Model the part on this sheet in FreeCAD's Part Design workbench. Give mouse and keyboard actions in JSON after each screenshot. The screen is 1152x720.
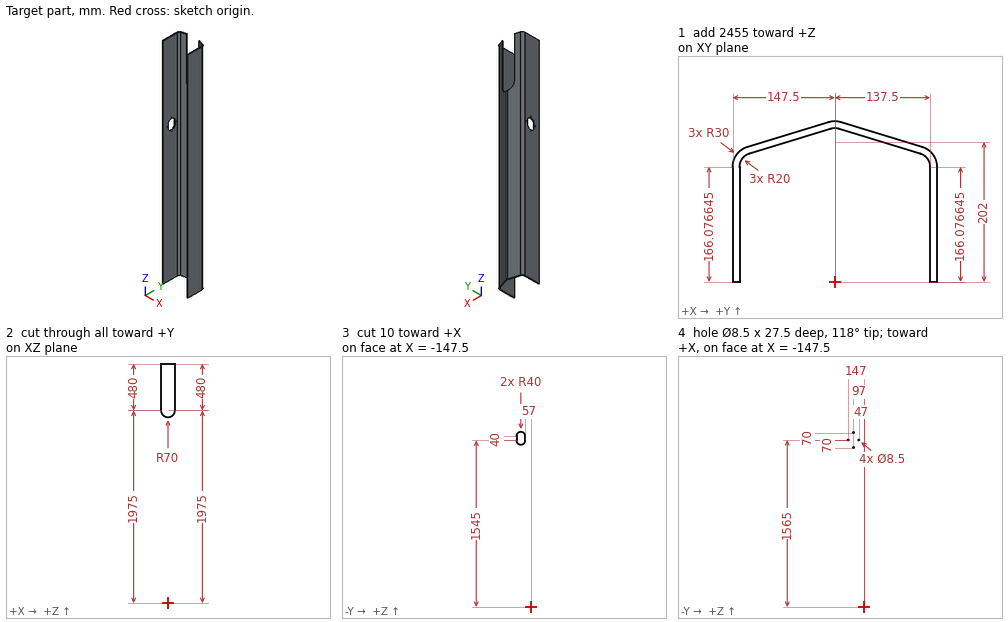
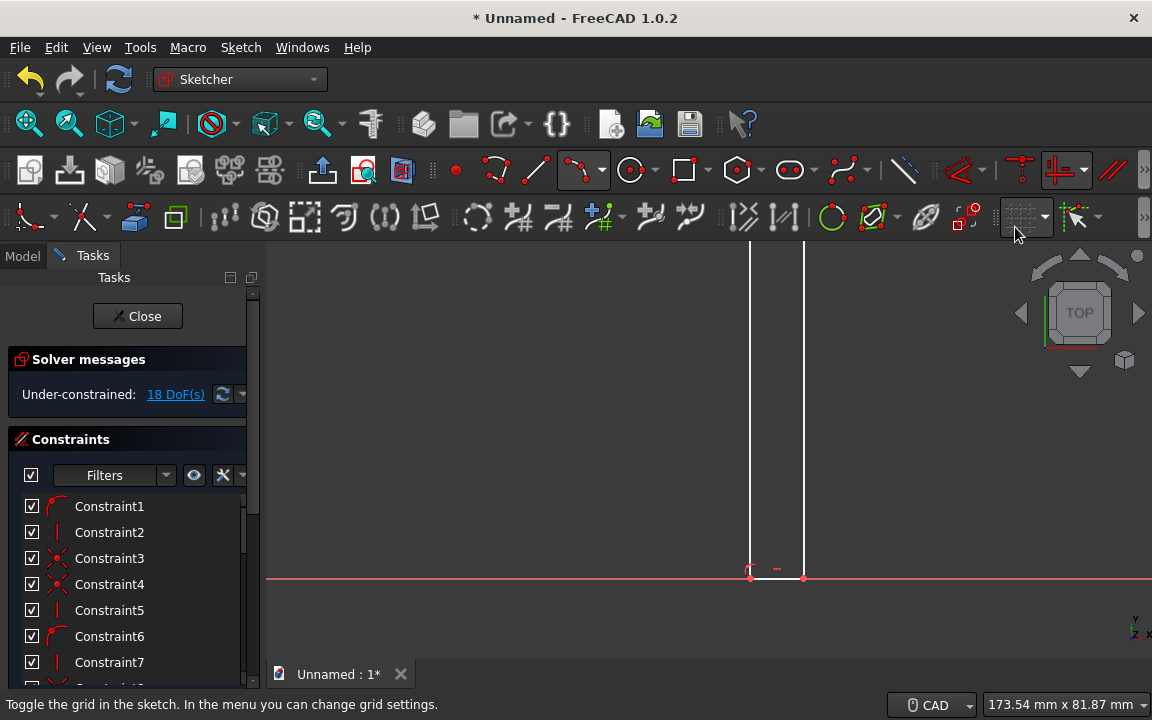
{"action": "scroll", "coordinate": [791, 567], "scroll_direction": "down", "scroll_amount": 8}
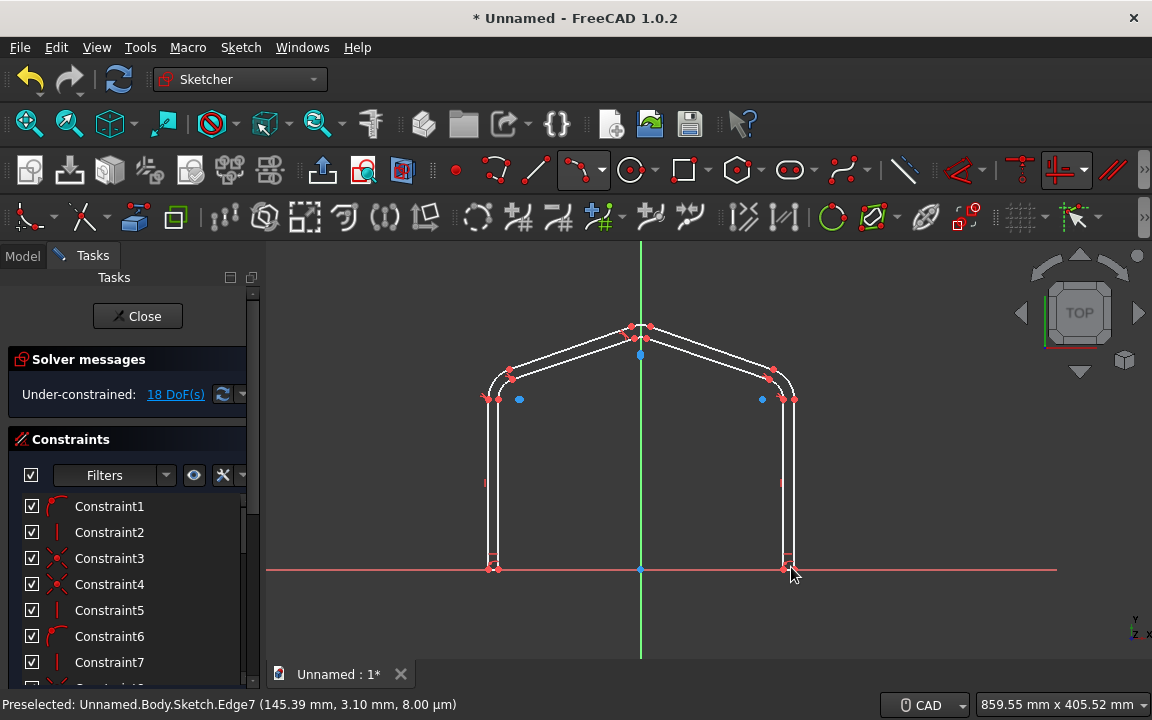
{"action": "scroll", "coordinate": [782, 392], "scroll_direction": "up", "scroll_amount": 3}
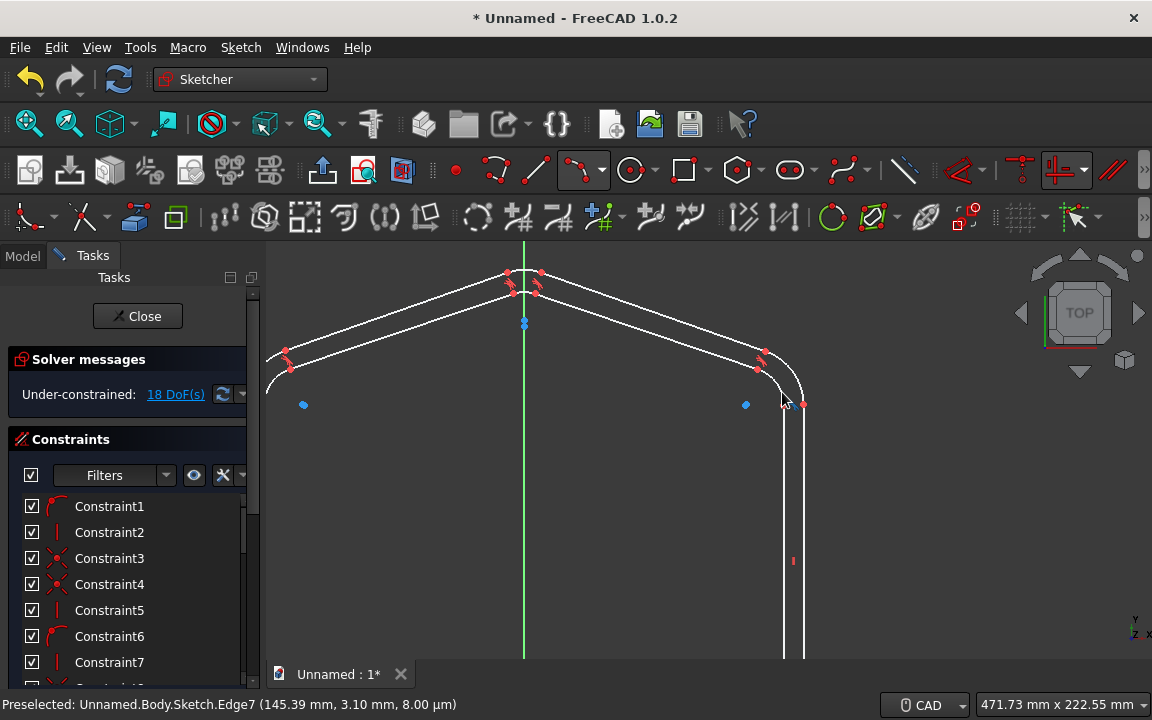
{"action": "left_click", "coordinate": [781, 392]}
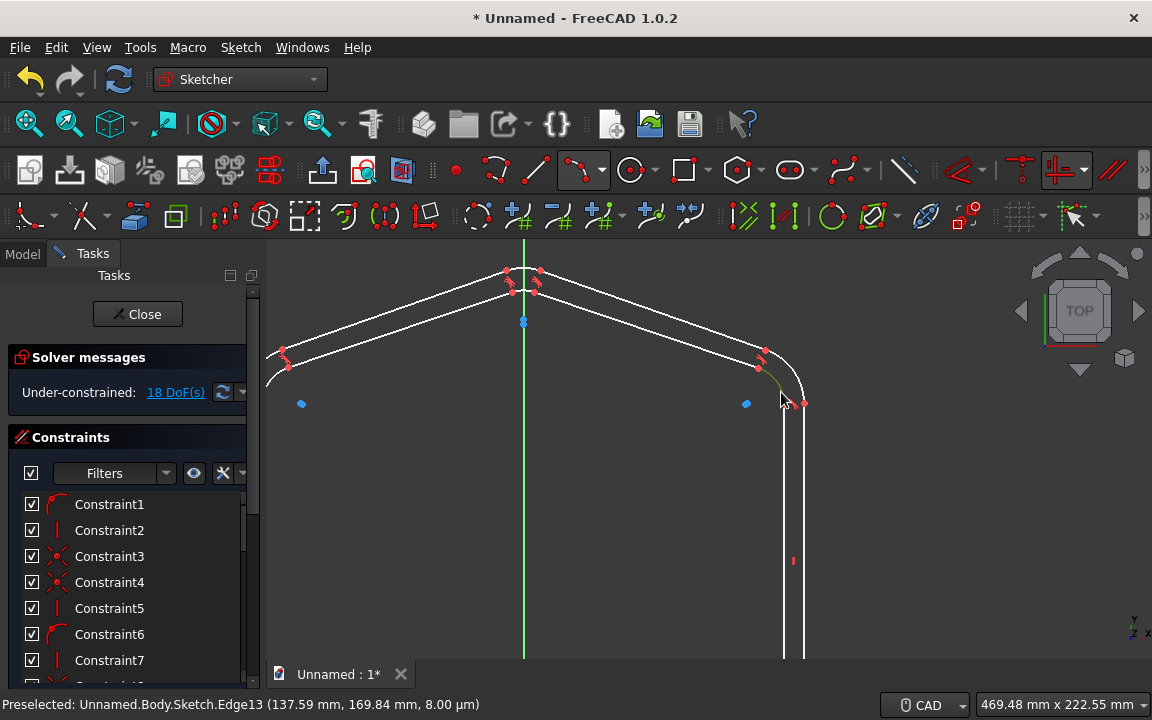
{"action": "left_click", "coordinate": [800, 383]}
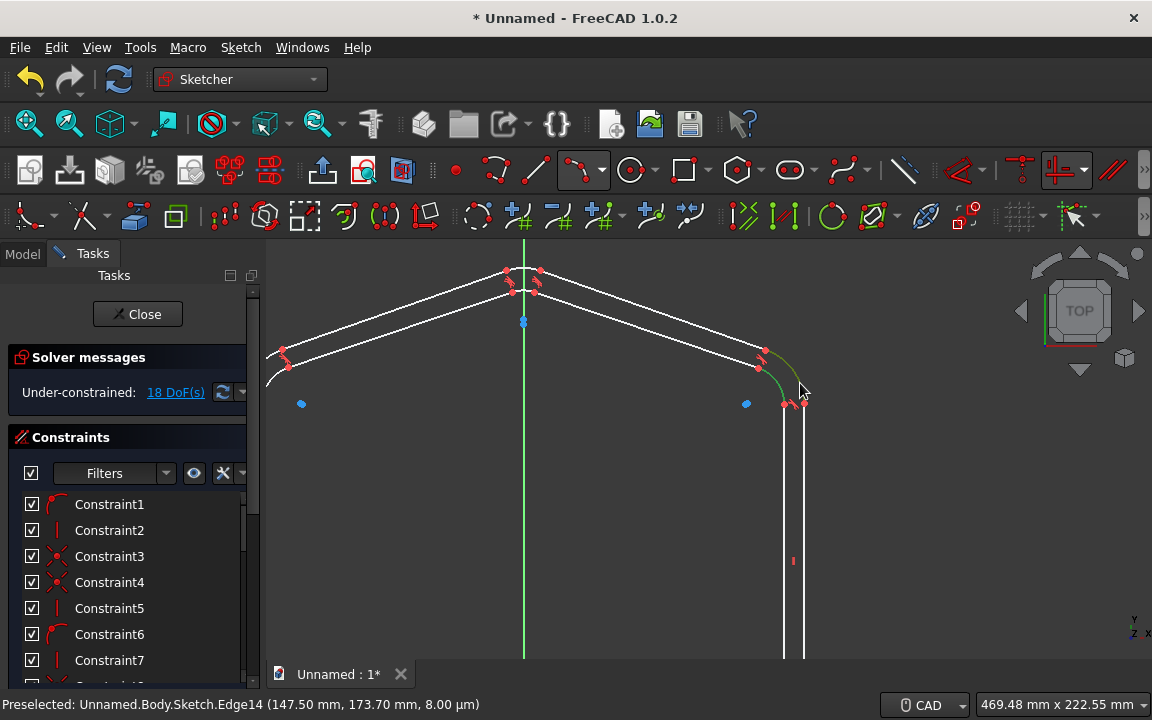
{"action": "left_click", "coordinate": [1020, 170]}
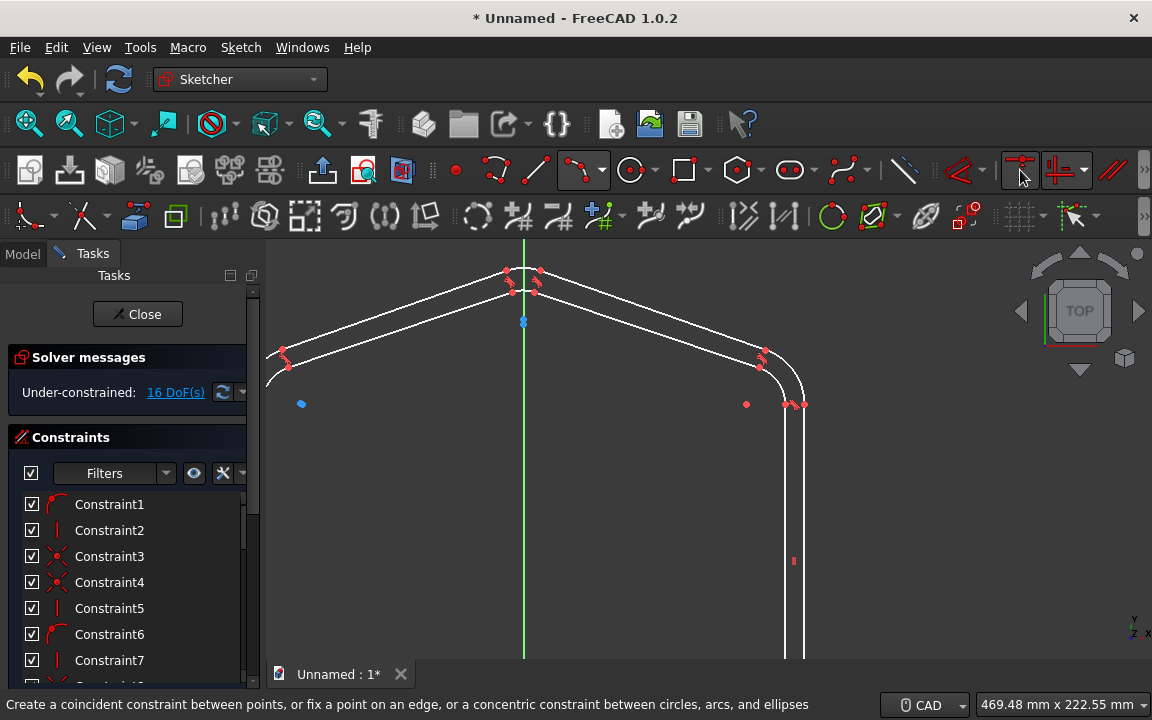
{"action": "scroll", "coordinate": [523, 290], "scroll_direction": "up", "scroll_amount": 2}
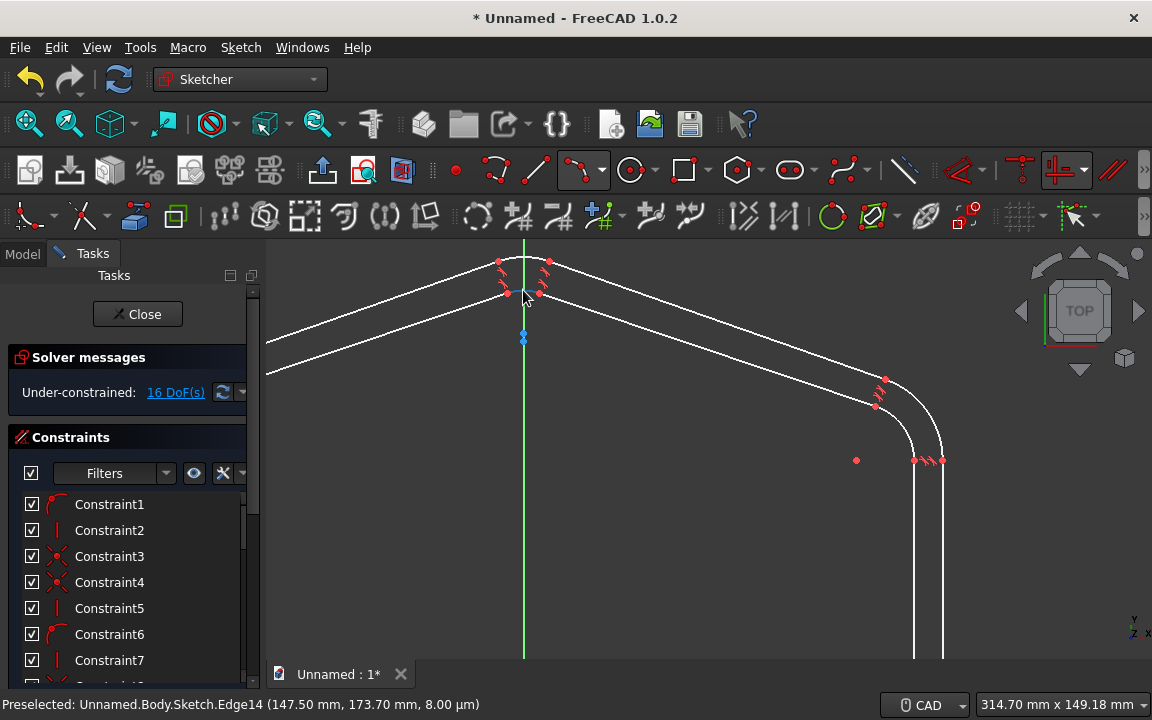
{"action": "left_click", "coordinate": [523, 291]}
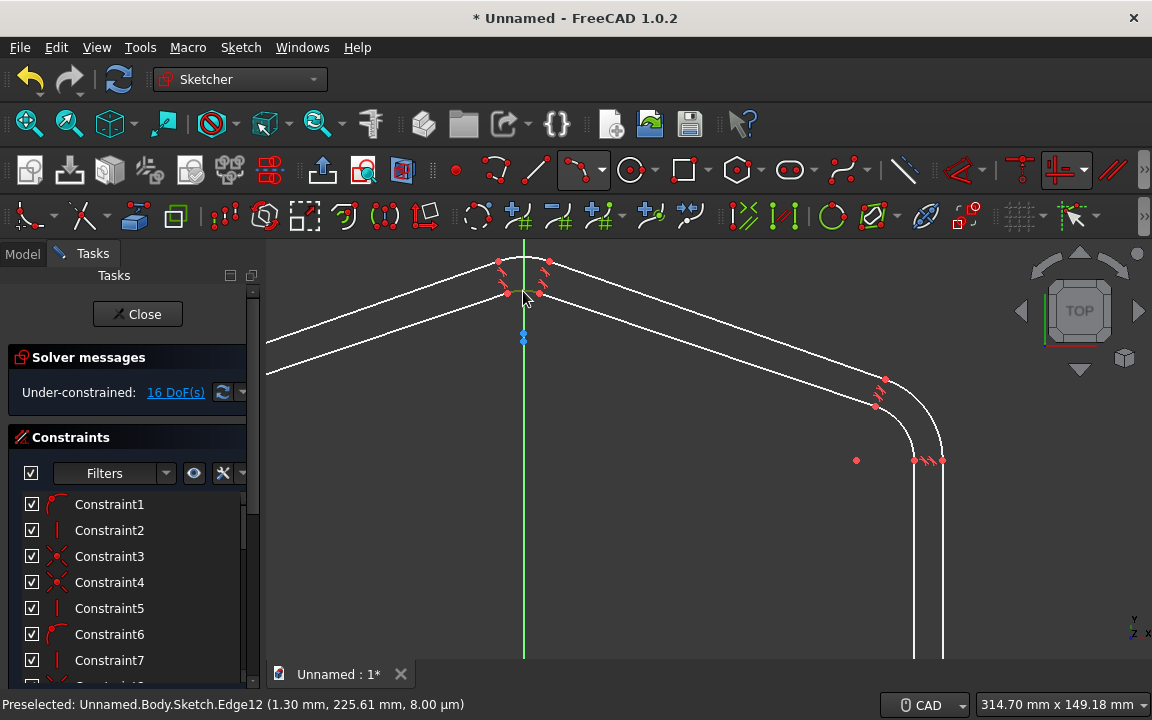
{"action": "scroll", "coordinate": [708, 362], "scroll_direction": "down", "scroll_amount": 5}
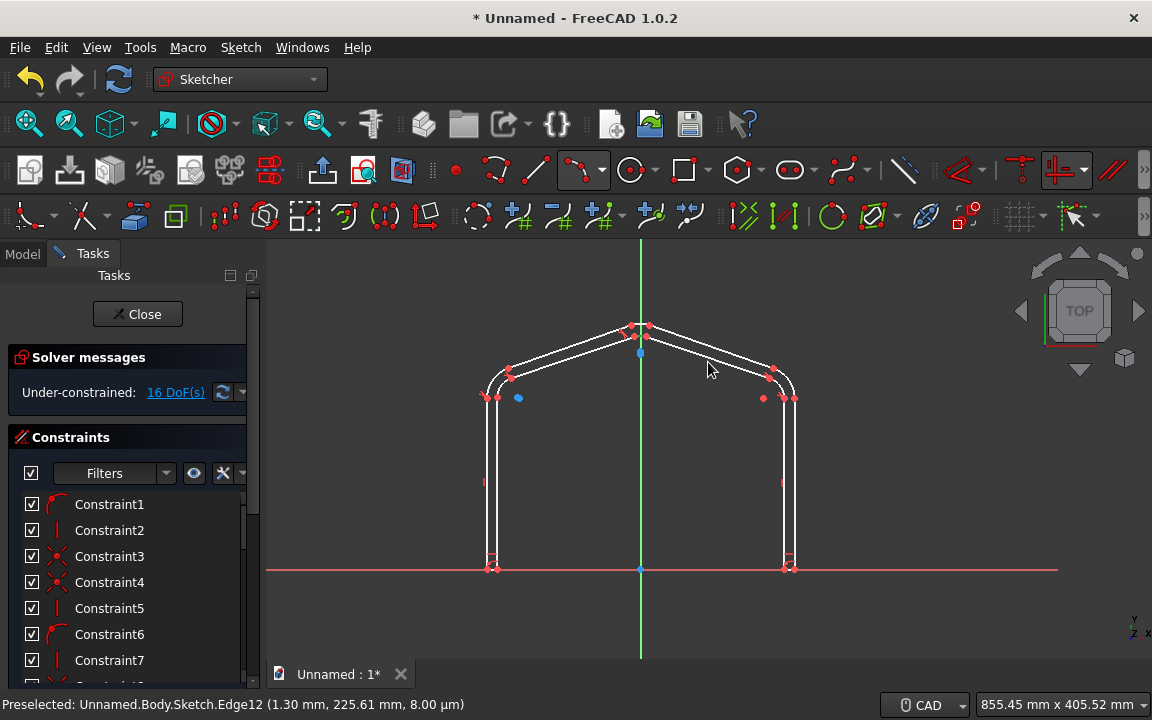
{"action": "scroll", "coordinate": [644, 324], "scroll_direction": "up", "scroll_amount": 7}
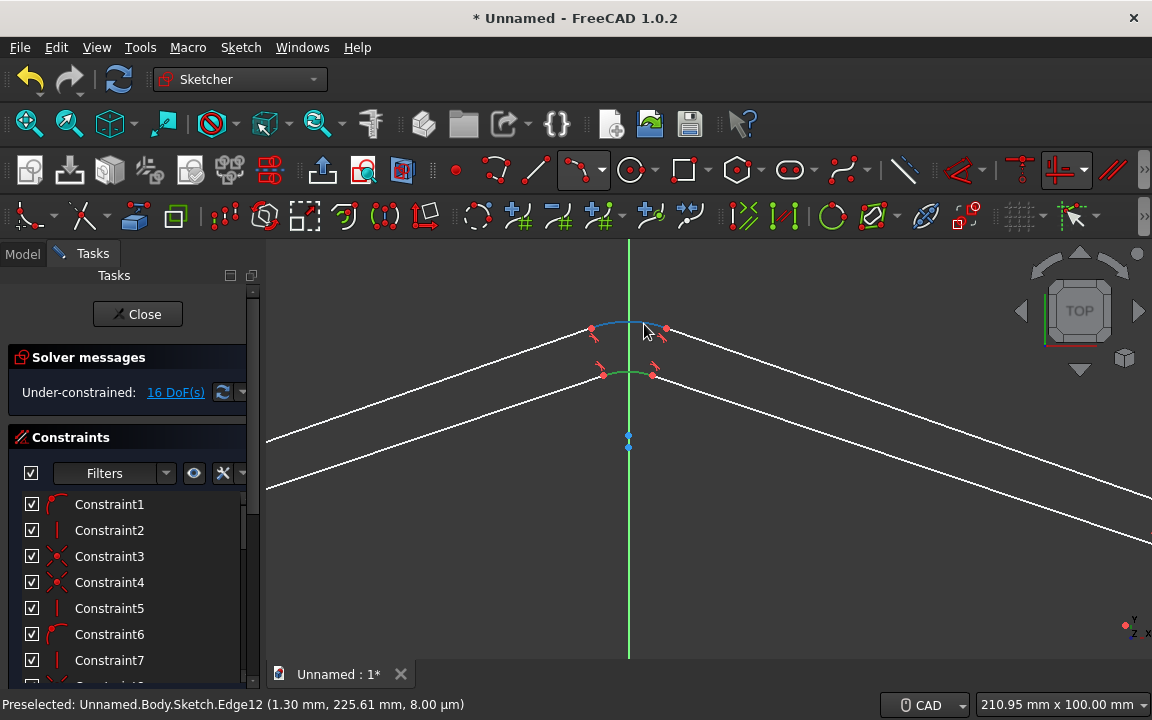
{"action": "left_click", "coordinate": [644, 323]}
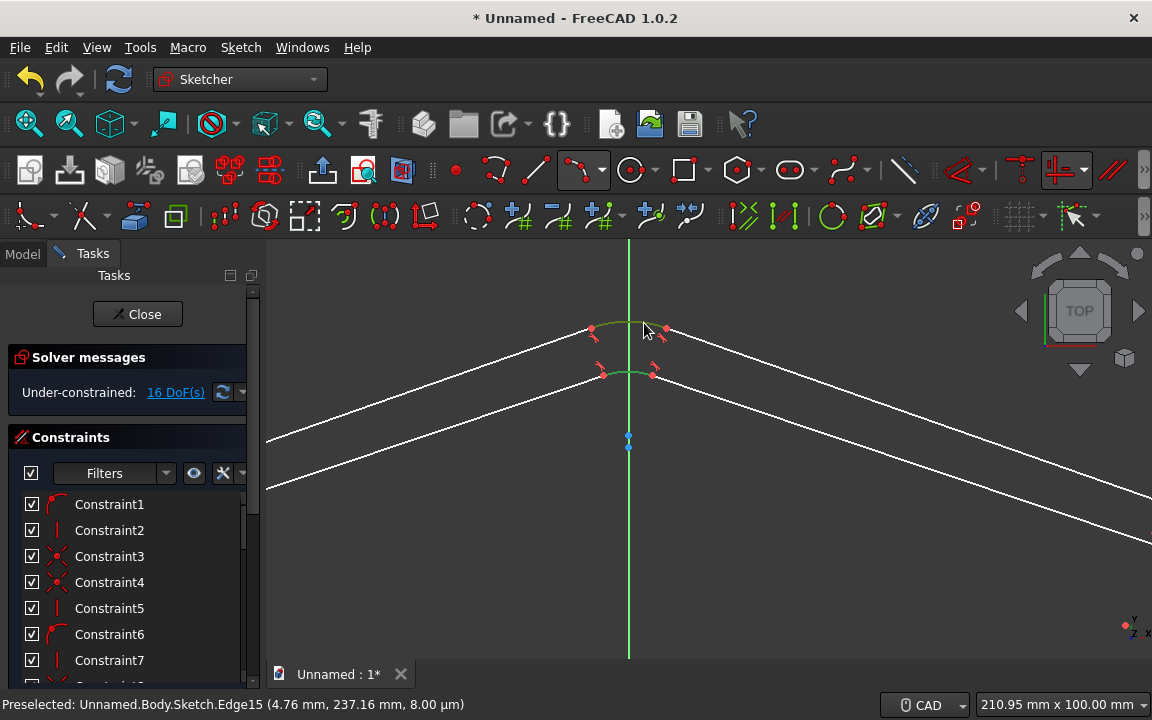
{"action": "left_click", "coordinate": [1020, 170]}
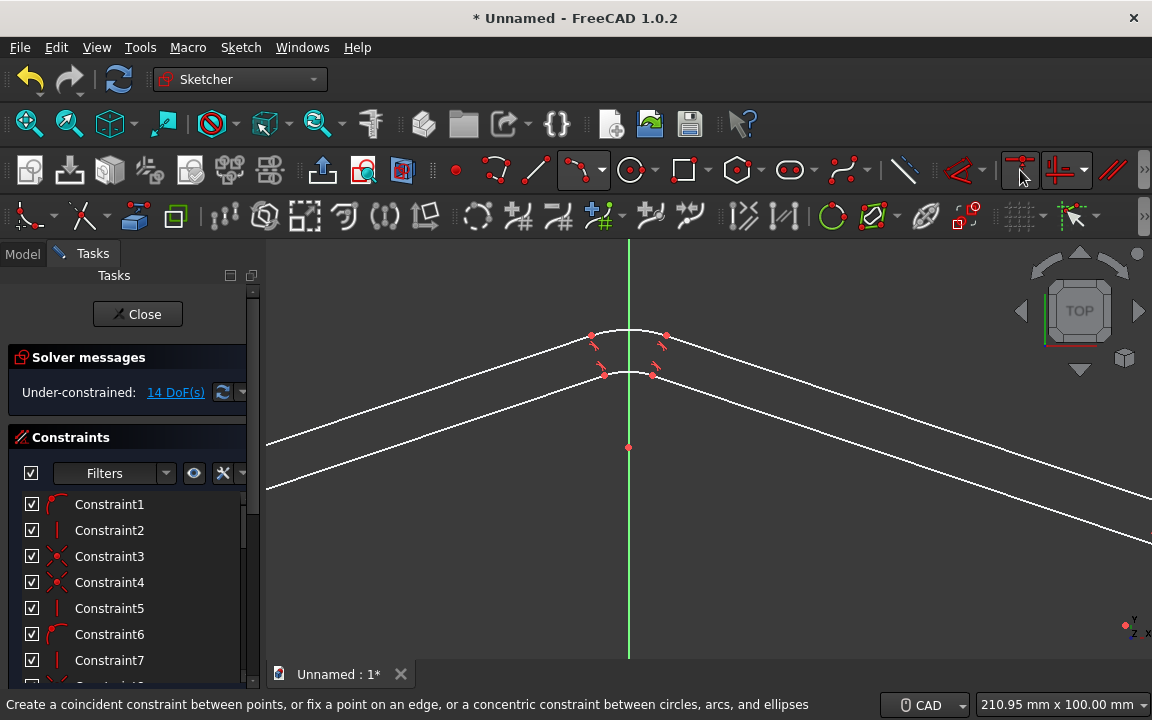
{"action": "scroll", "coordinate": [644, 324], "scroll_direction": "down", "scroll_amount": 7}